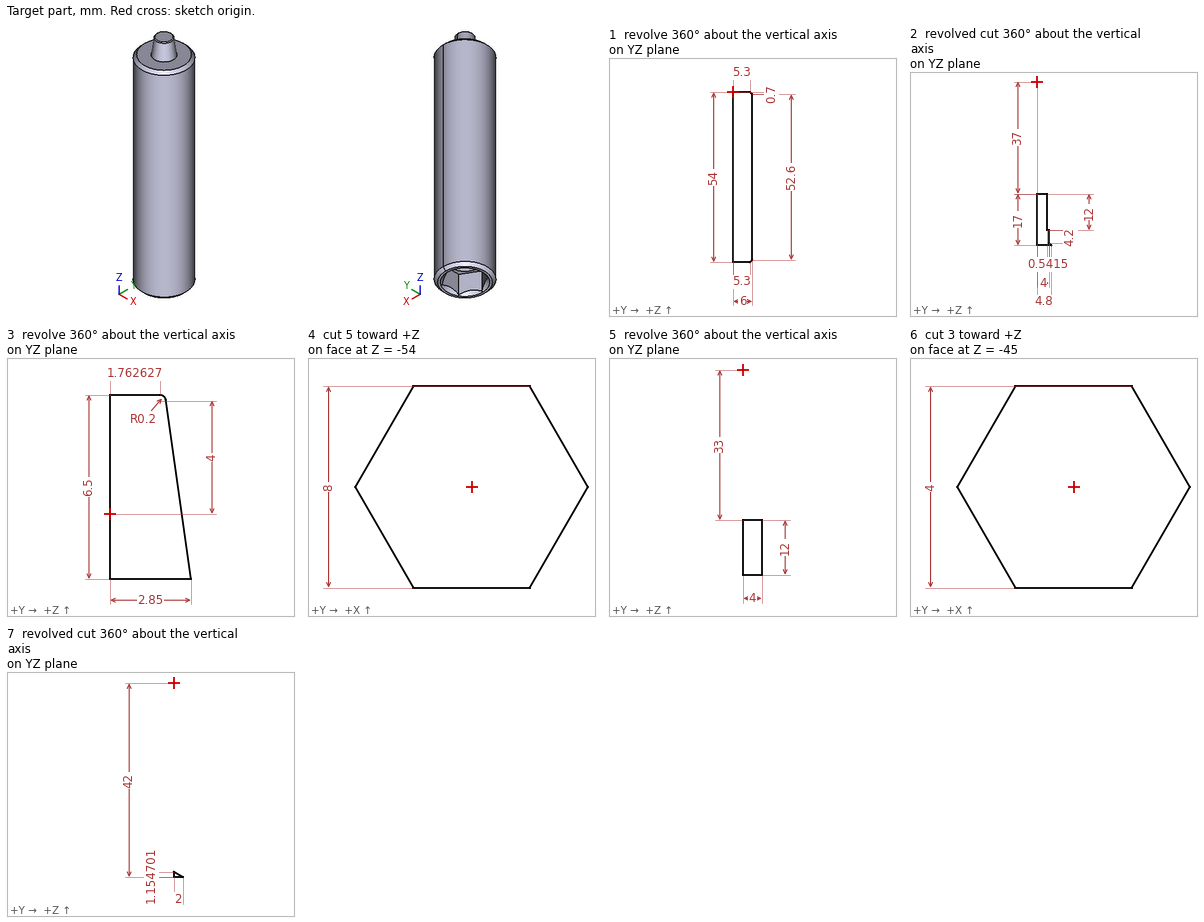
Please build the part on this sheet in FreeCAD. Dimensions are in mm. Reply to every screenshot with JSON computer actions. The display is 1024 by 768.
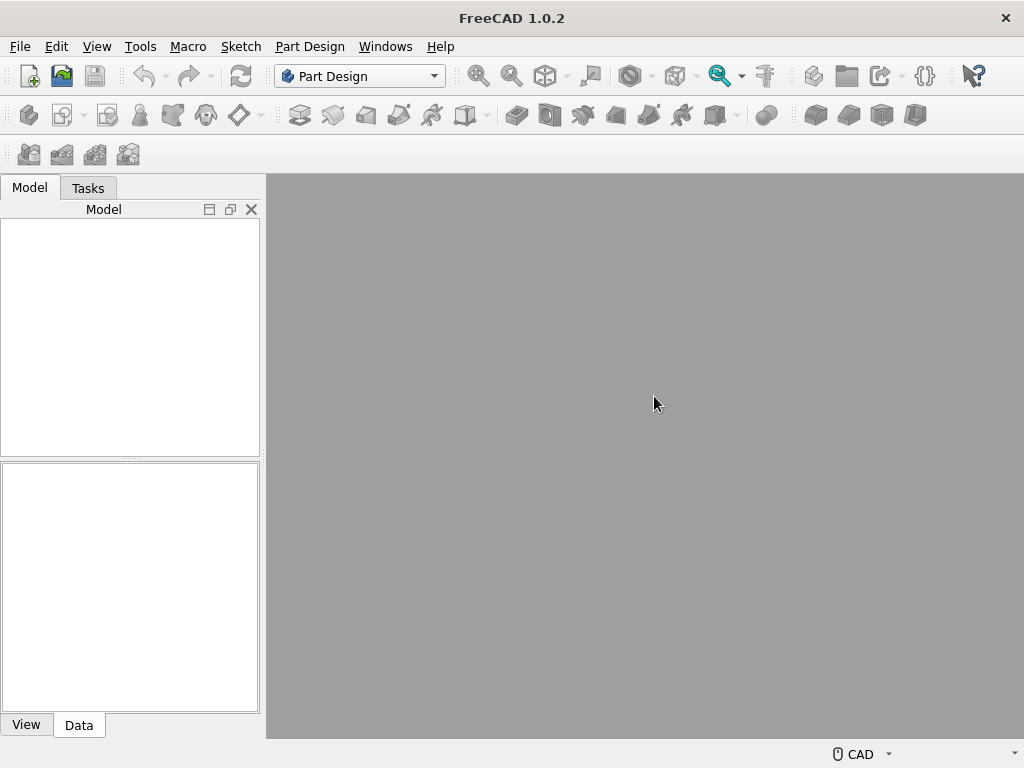
{"action": "left_click", "coordinate": [29, 76]}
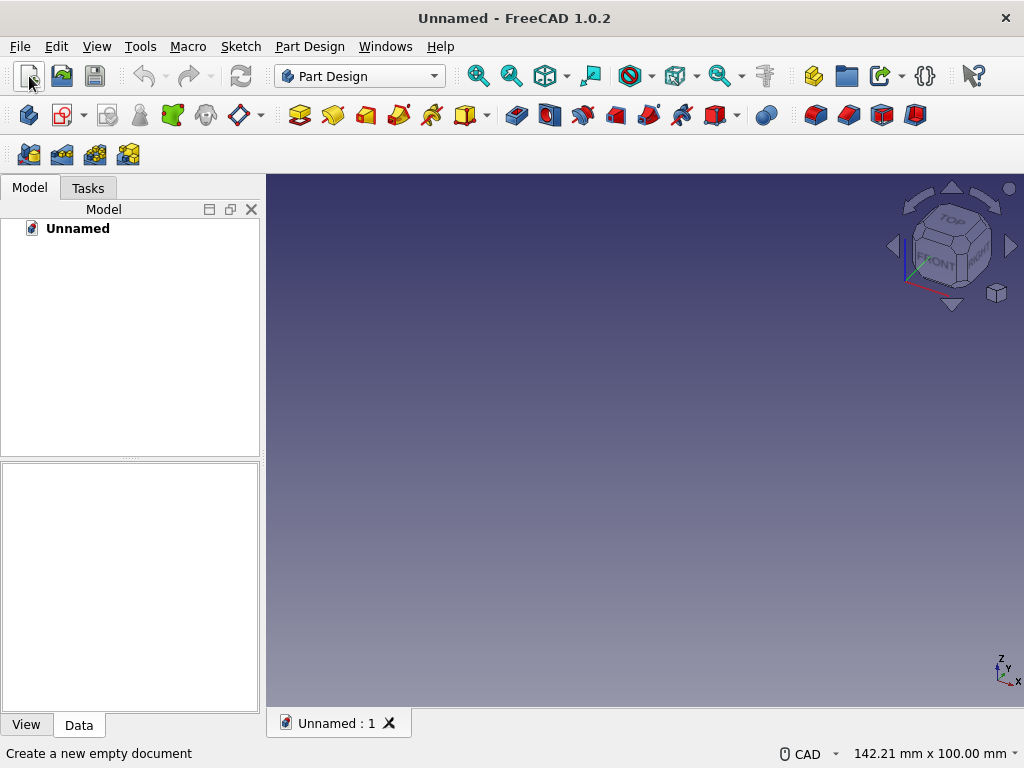
{"action": "left_click", "coordinate": [62, 116]}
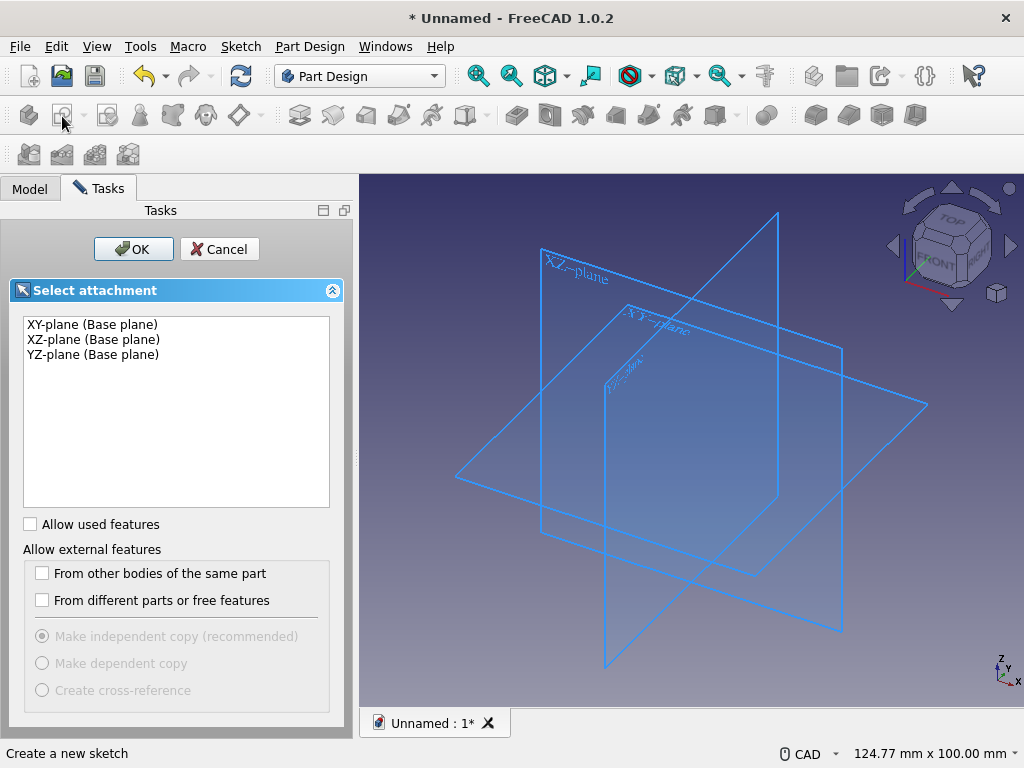
{"action": "left_click", "coordinate": [84, 354]}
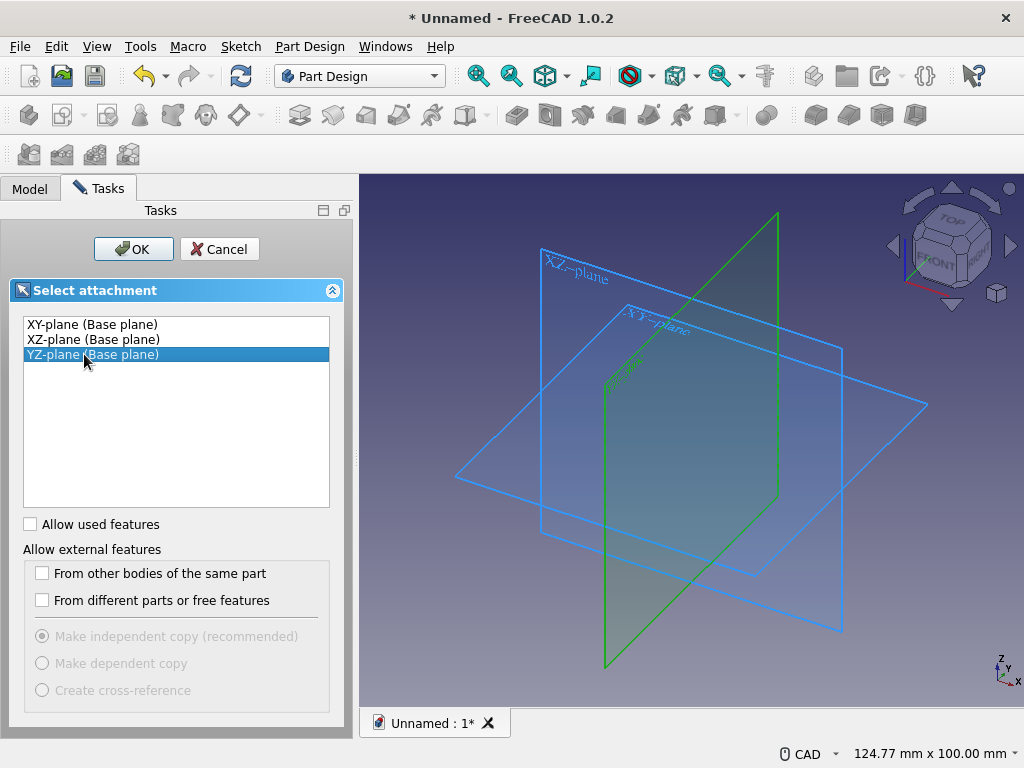
{"action": "left_click", "coordinate": [134, 249]}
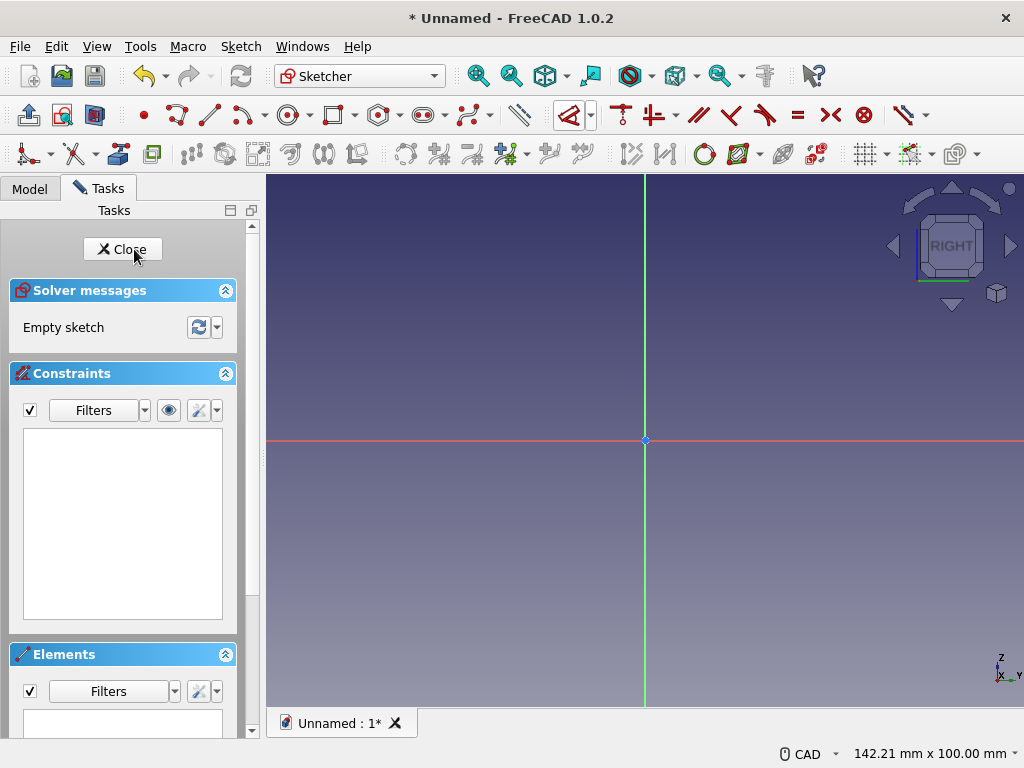
{"action": "scroll", "coordinate": [294, 202], "scroll_direction": "down", "scroll_amount": 1}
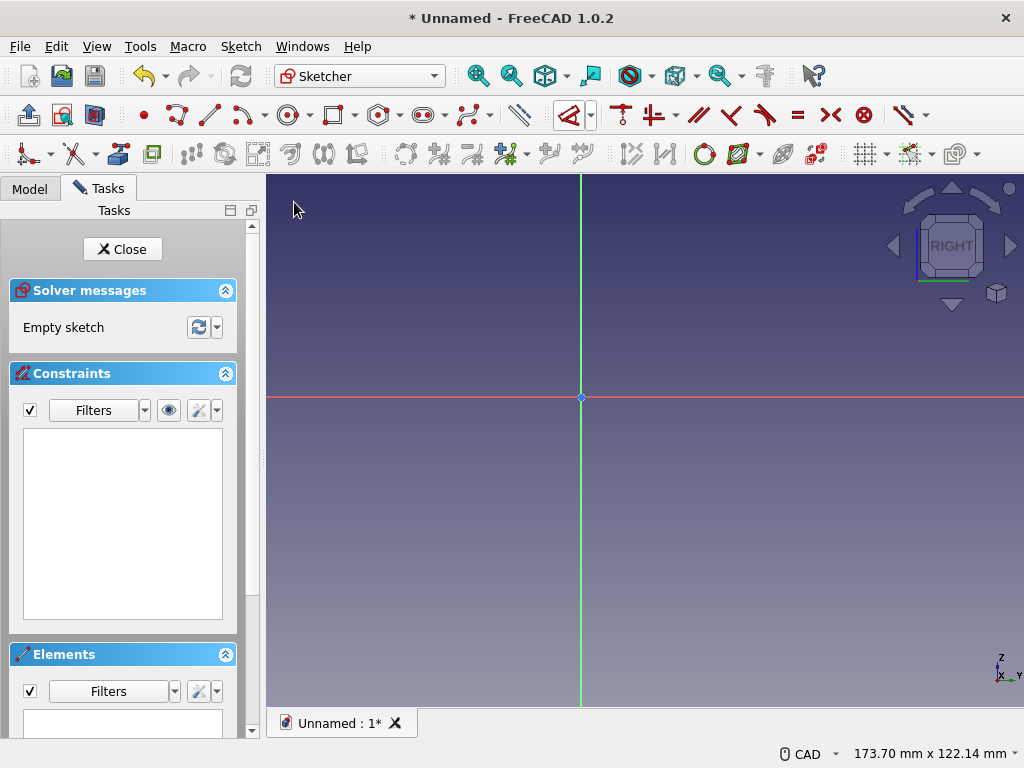
{"action": "scroll", "coordinate": [631, 667], "scroll_direction": "up", "scroll_amount": 2}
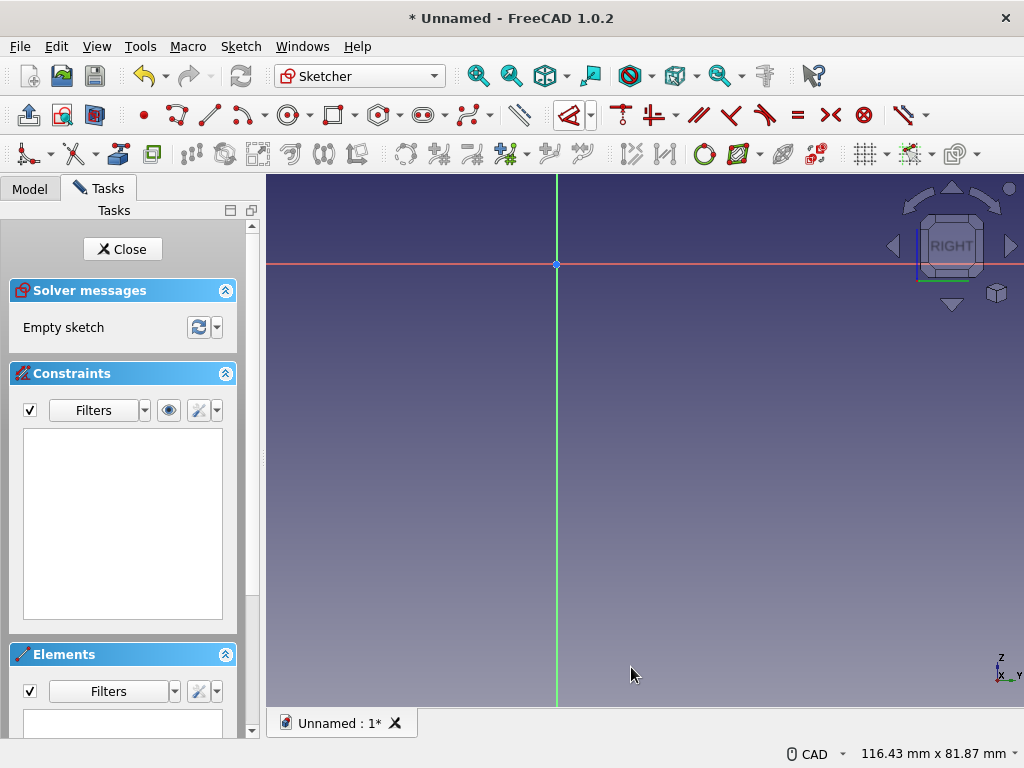
{"action": "left_click", "coordinate": [177, 116]}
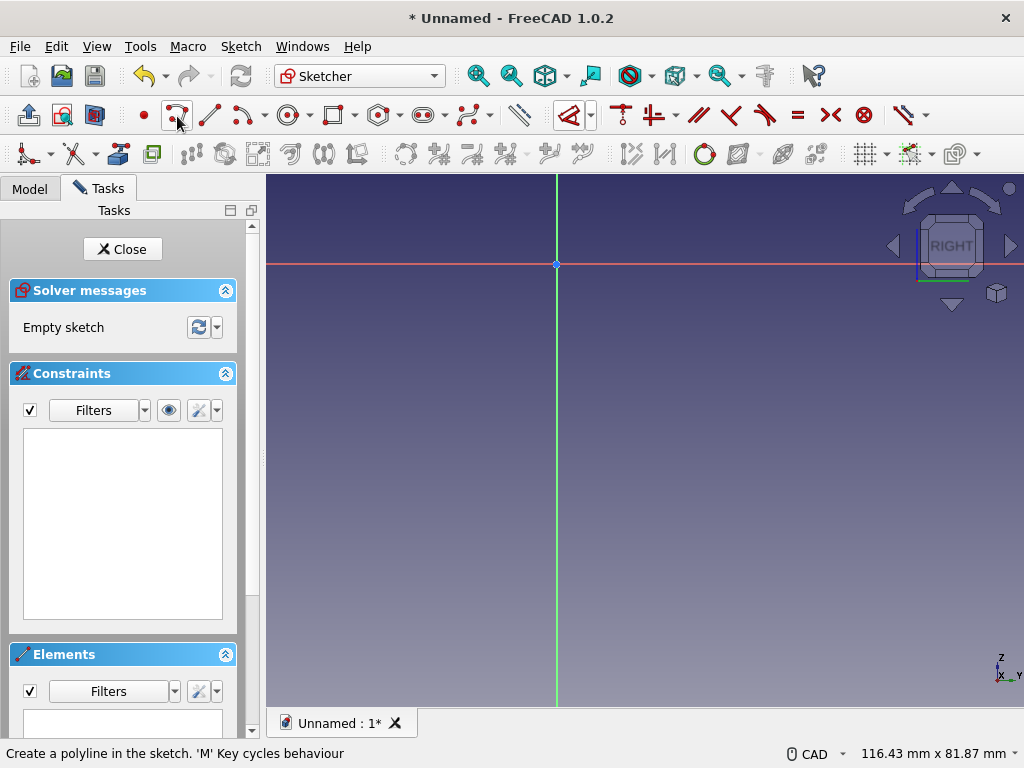
{"action": "left_click", "coordinate": [557, 264]}
{"action": "left_click", "coordinate": [566, 616]}
{"action": "left_click", "coordinate": [591, 616]}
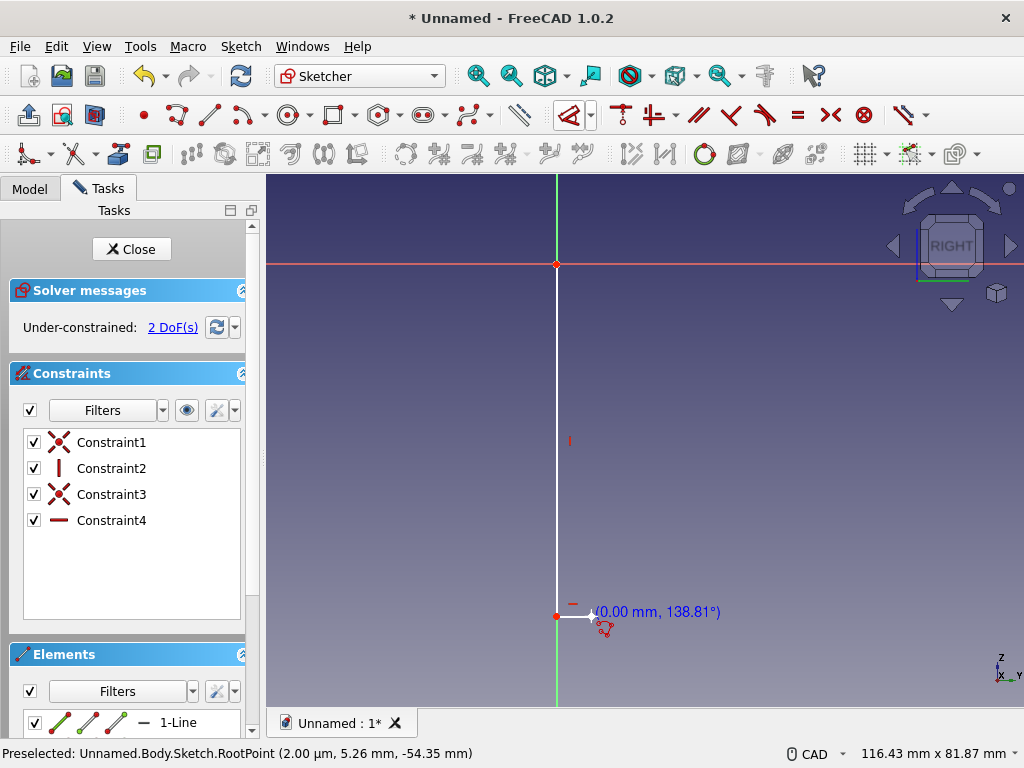
{"action": "scroll", "coordinate": [596, 611], "scroll_direction": "up", "scroll_amount": 5}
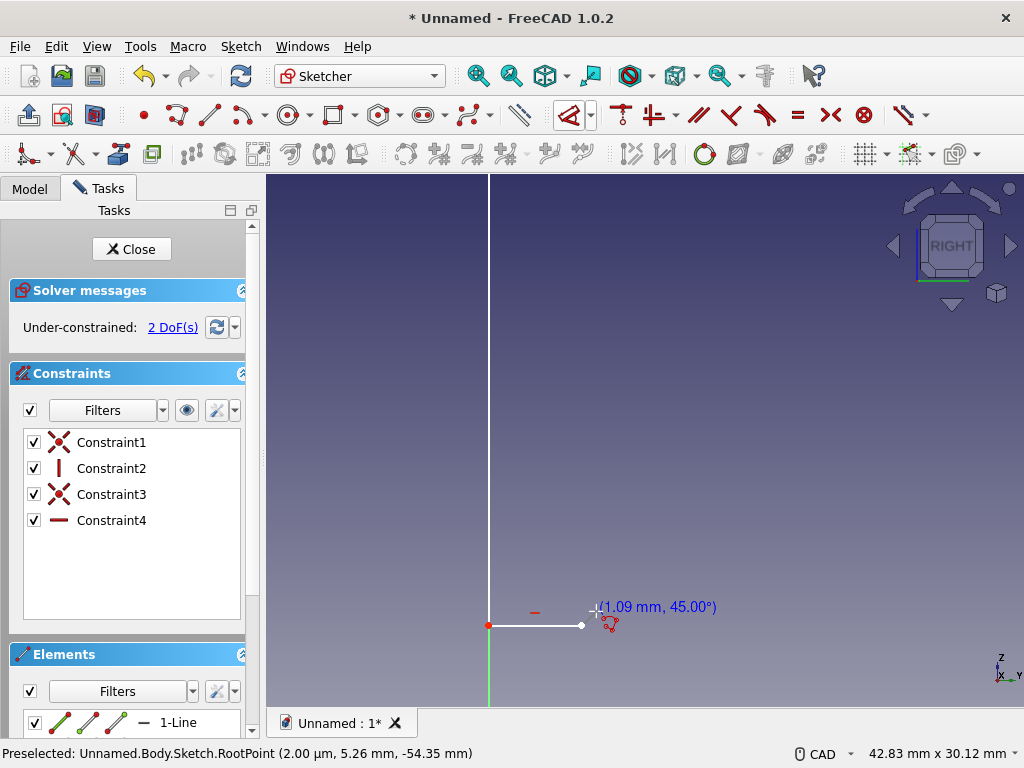
{"action": "left_click", "coordinate": [595, 610]}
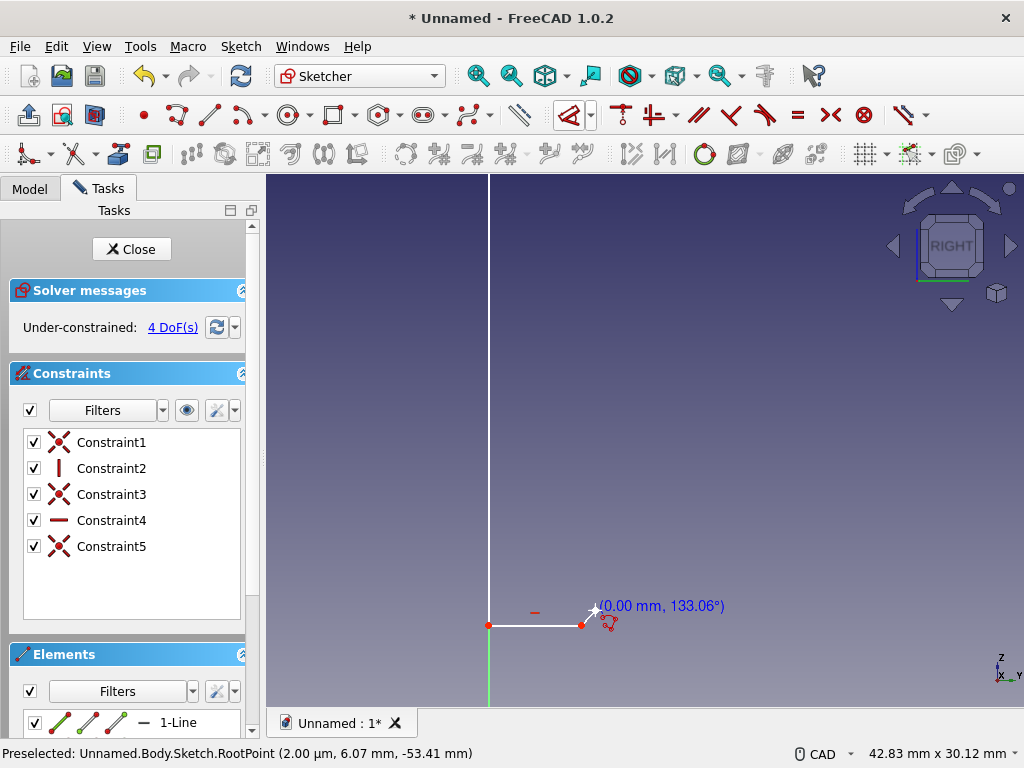
{"action": "scroll", "coordinate": [597, 613], "scroll_direction": "down", "scroll_amount": 5}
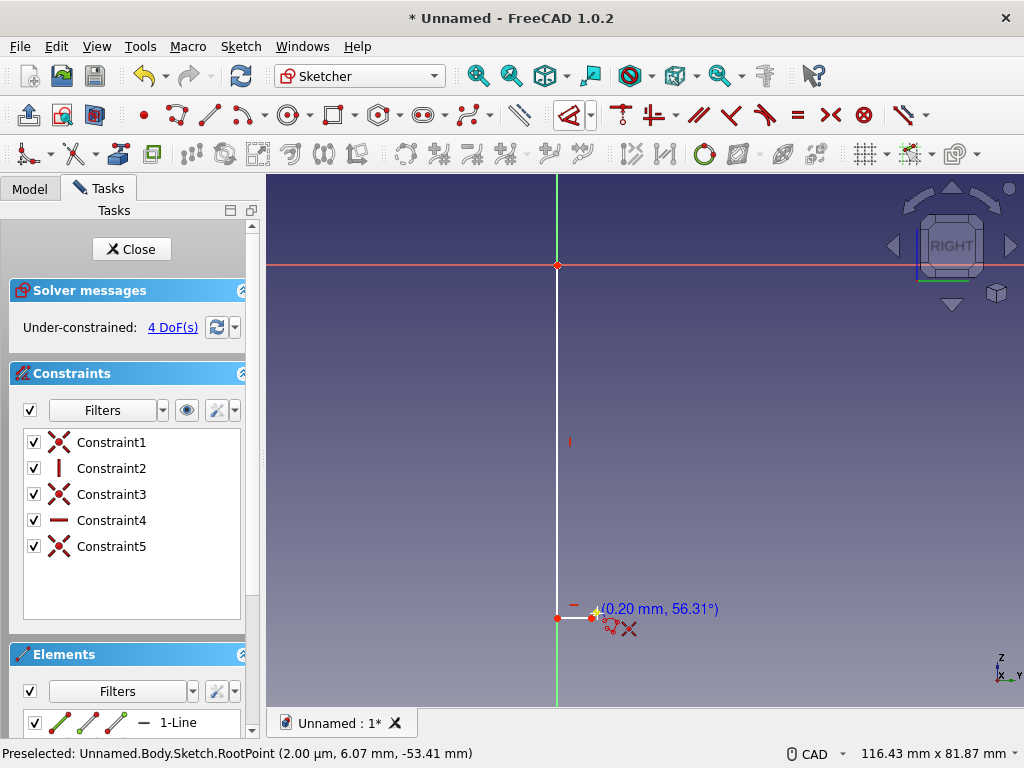
{"action": "scroll", "coordinate": [596, 270], "scroll_direction": "up", "scroll_amount": 7}